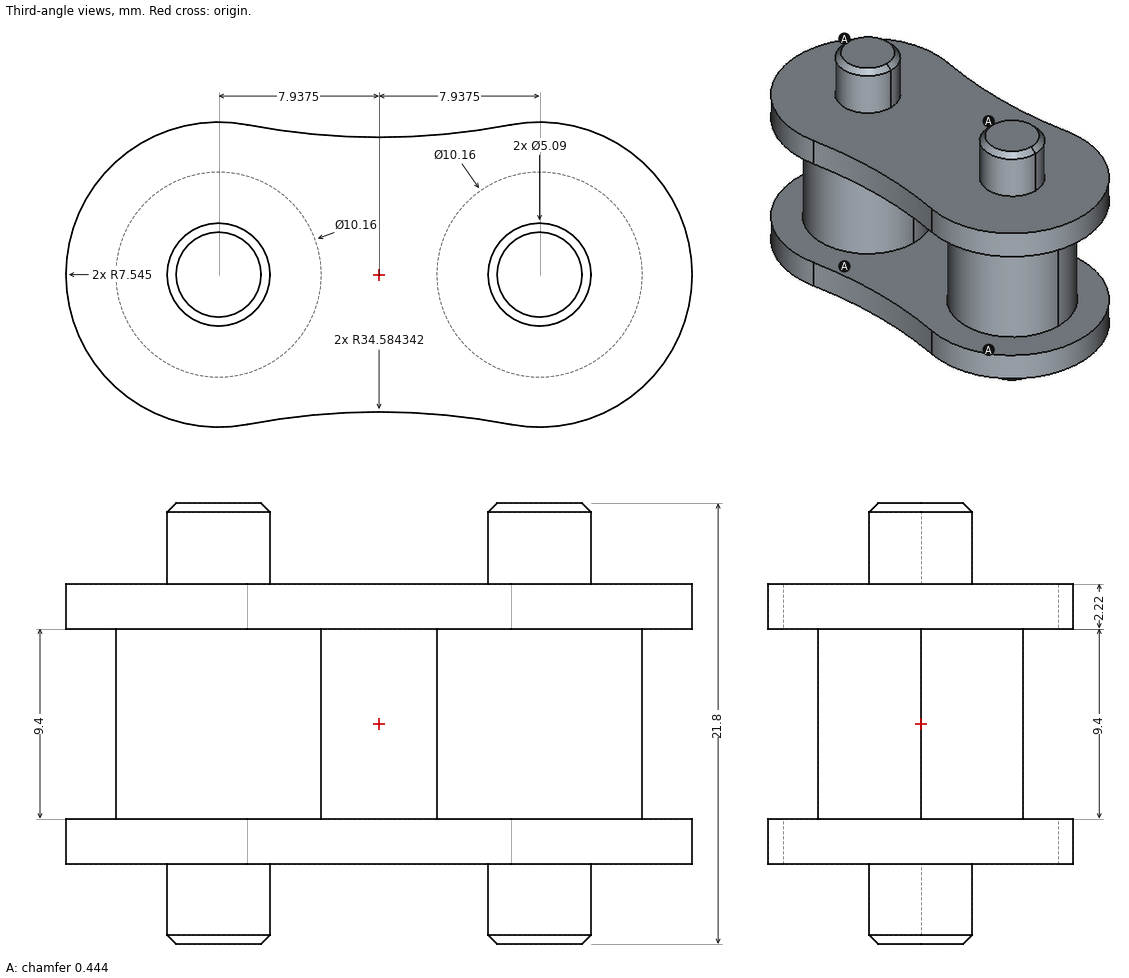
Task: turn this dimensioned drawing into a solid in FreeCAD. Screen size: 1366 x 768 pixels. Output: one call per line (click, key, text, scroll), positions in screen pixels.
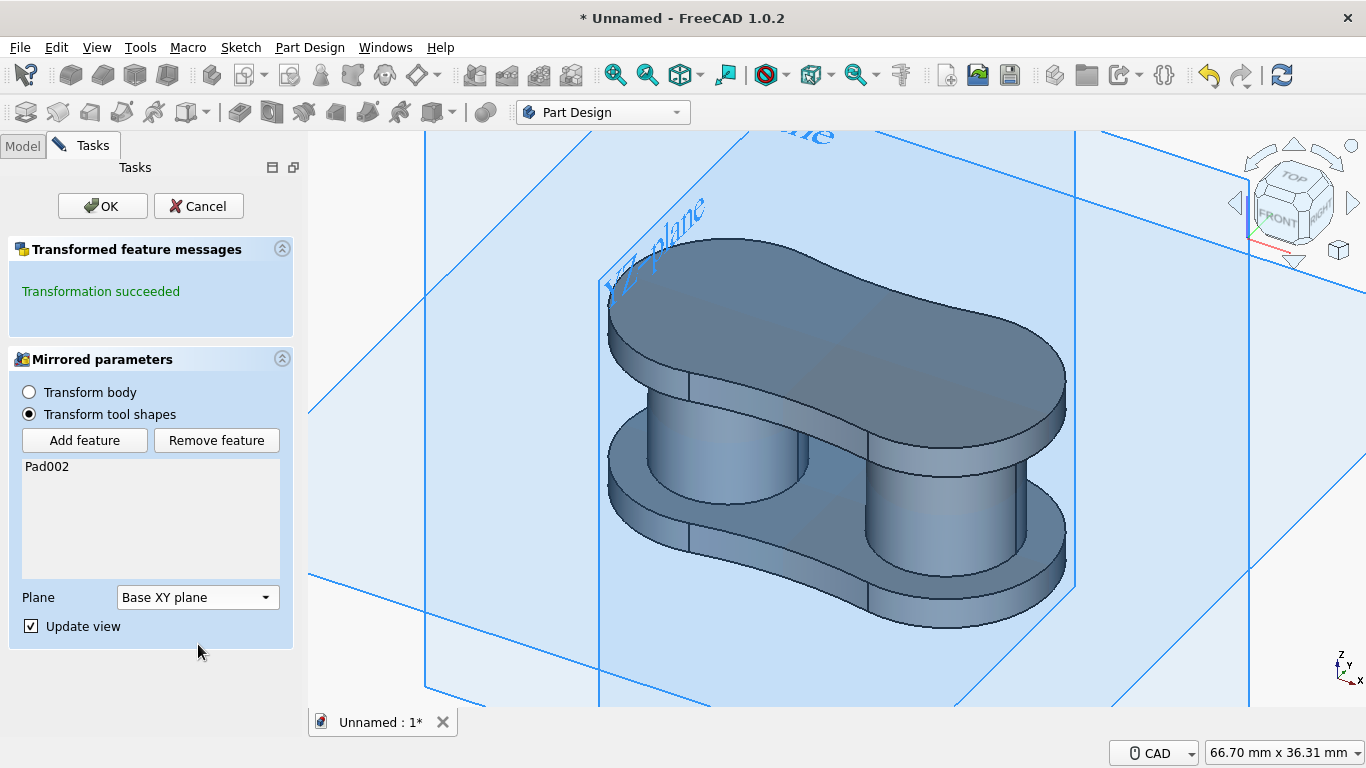
click(103, 206)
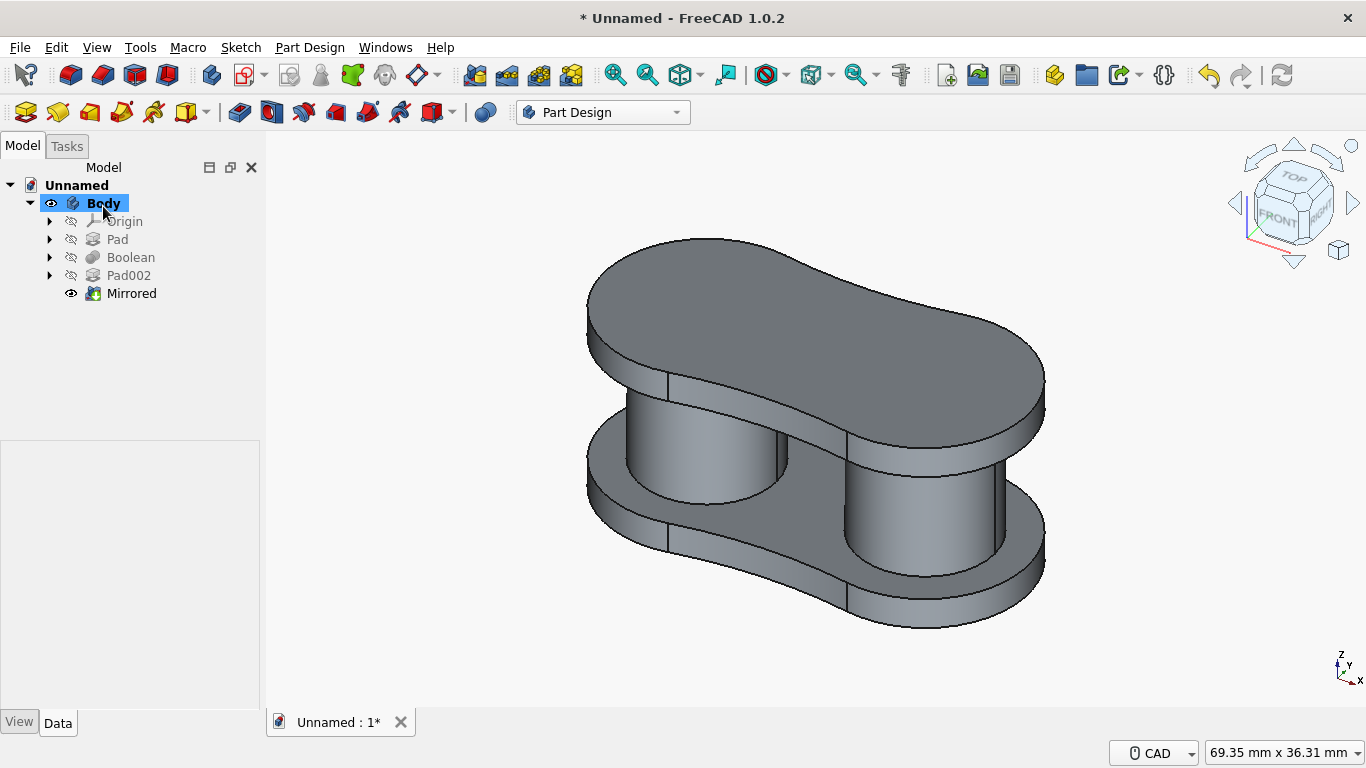
click(244, 76)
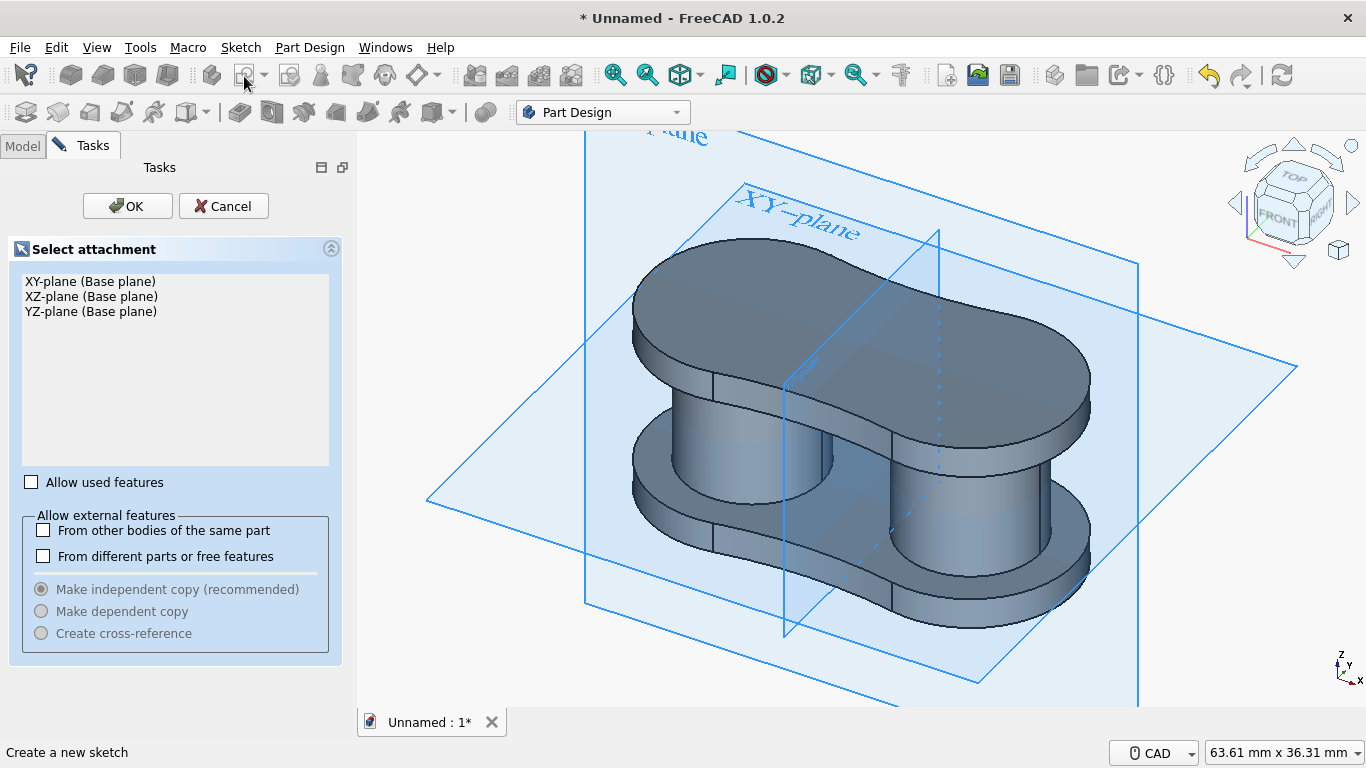
click(82, 282)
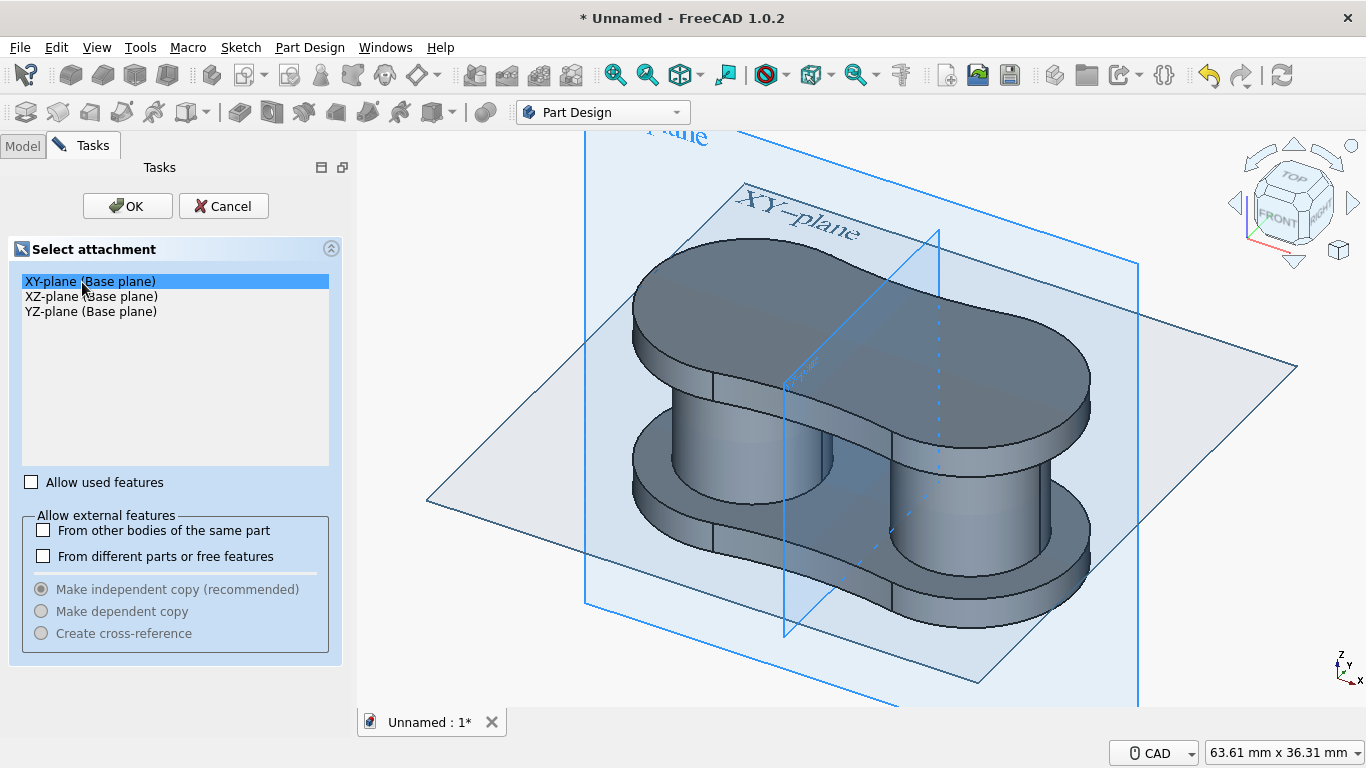
click(128, 206)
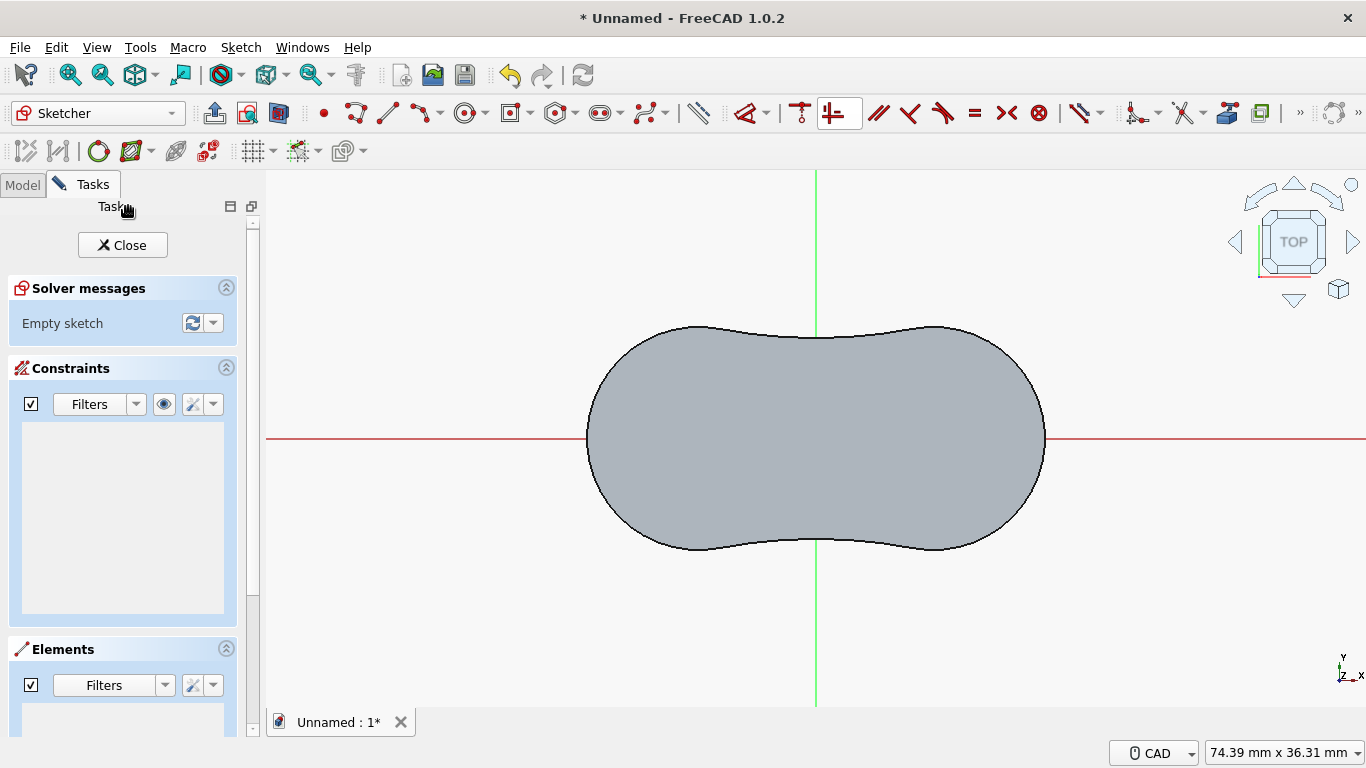
key(q)
key(s)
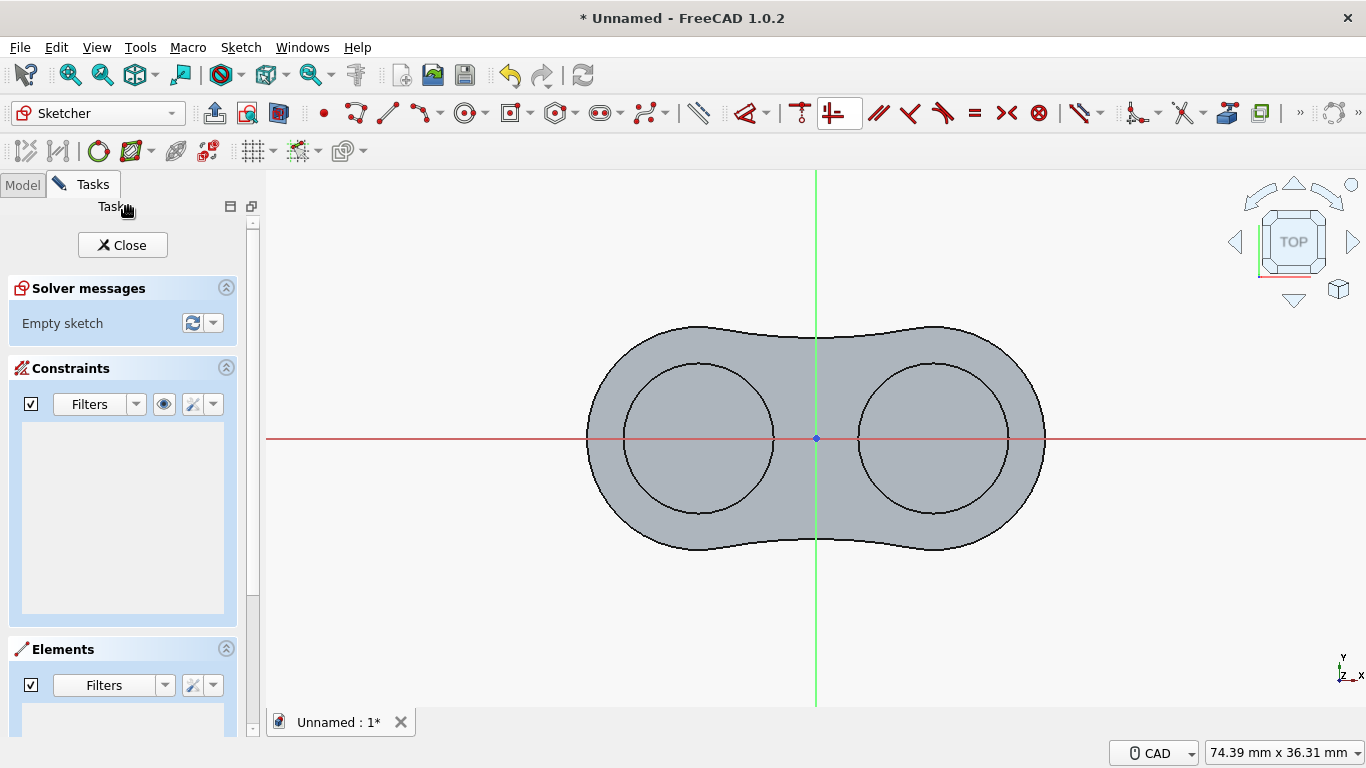
scroll(872, 438, up, 4)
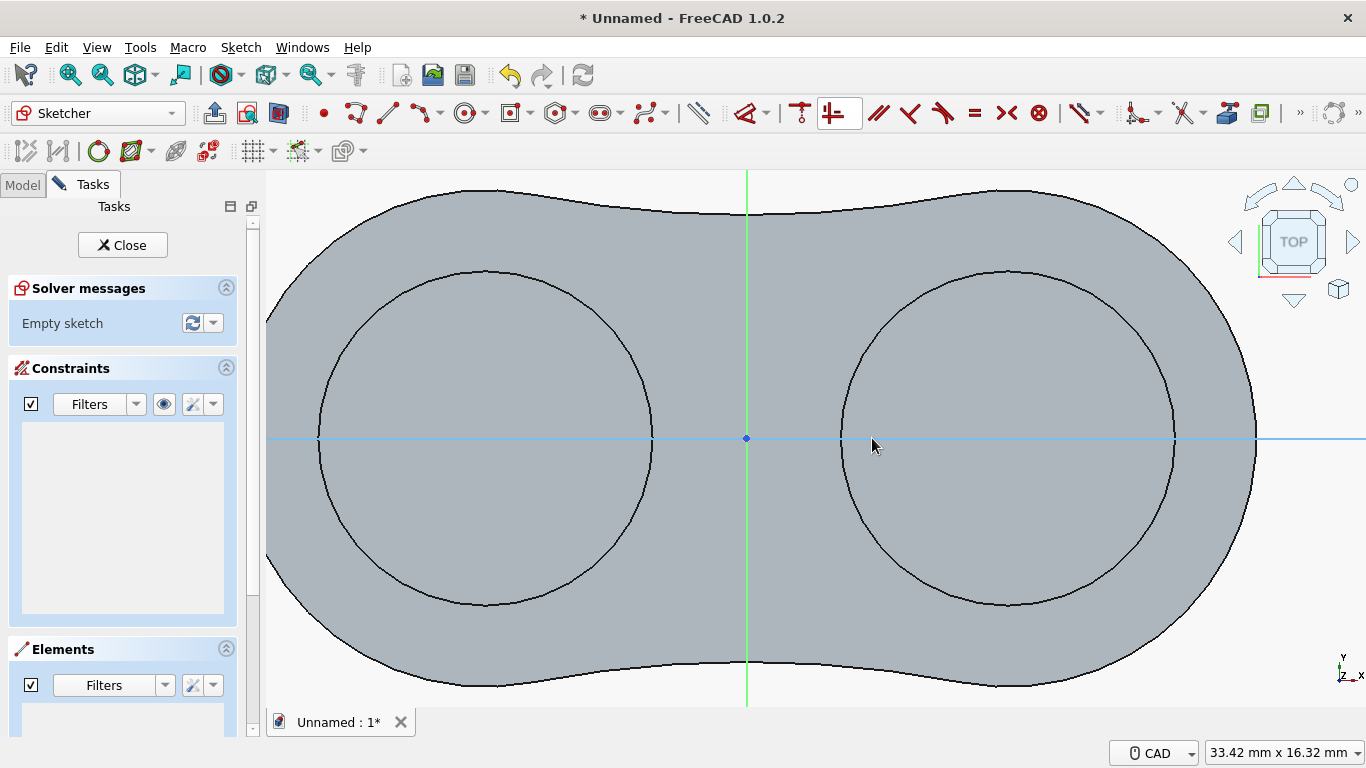
key(g)
key(c)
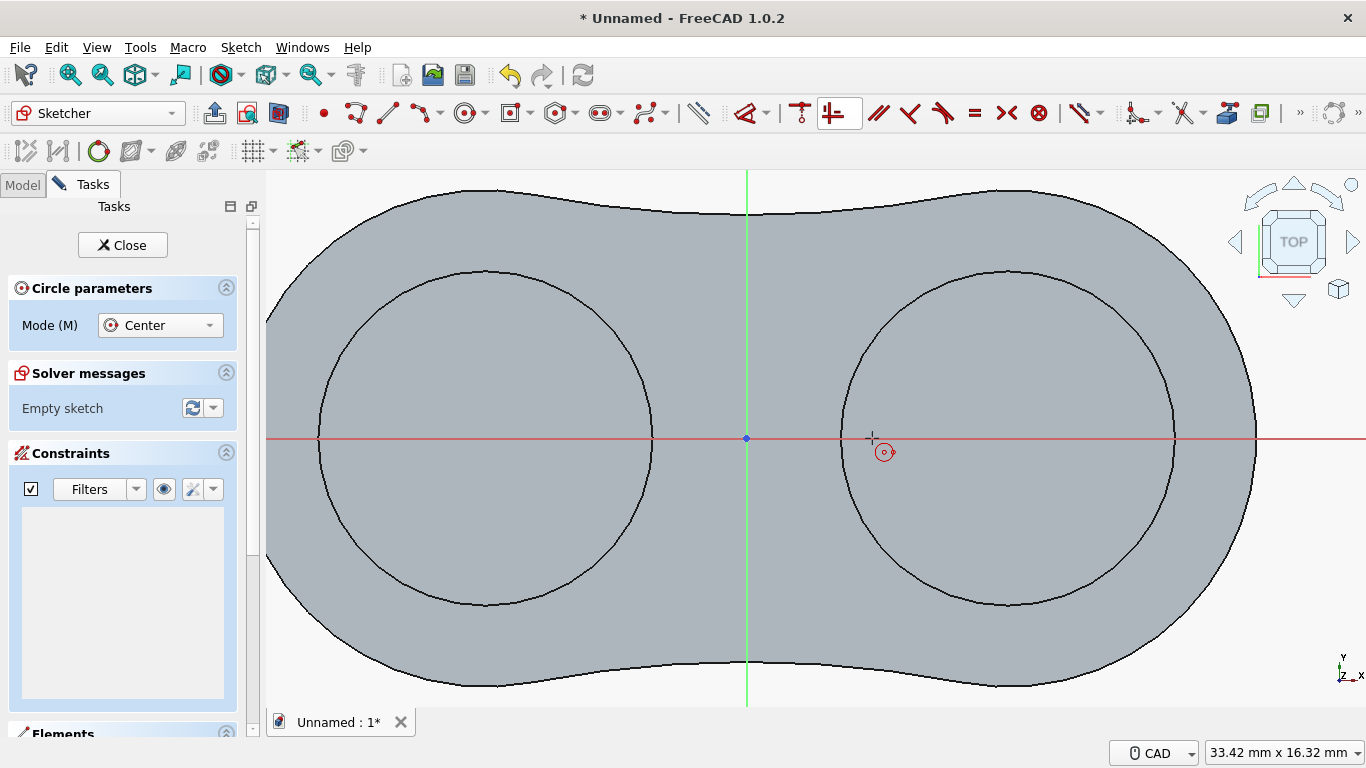
click(1008, 438)
move(1067, 379)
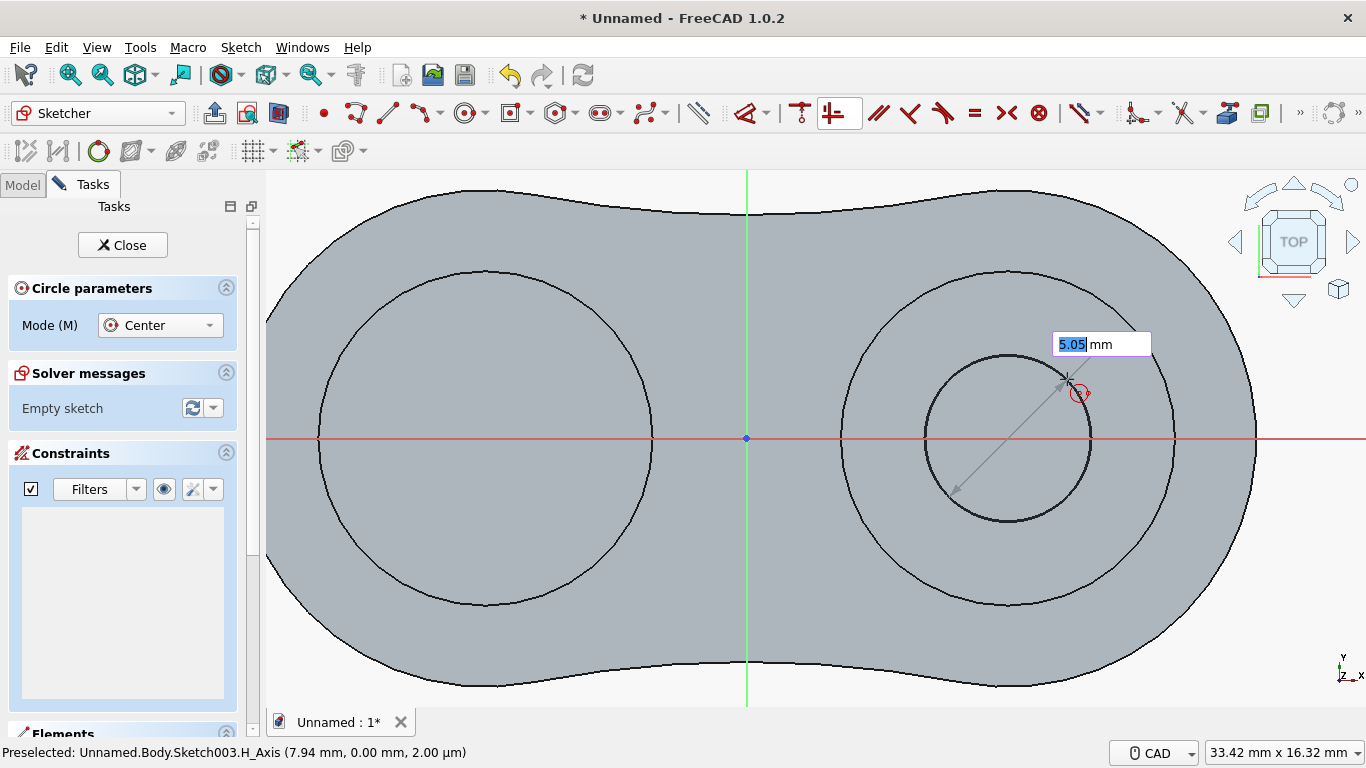
text(5.09)
key(Return)